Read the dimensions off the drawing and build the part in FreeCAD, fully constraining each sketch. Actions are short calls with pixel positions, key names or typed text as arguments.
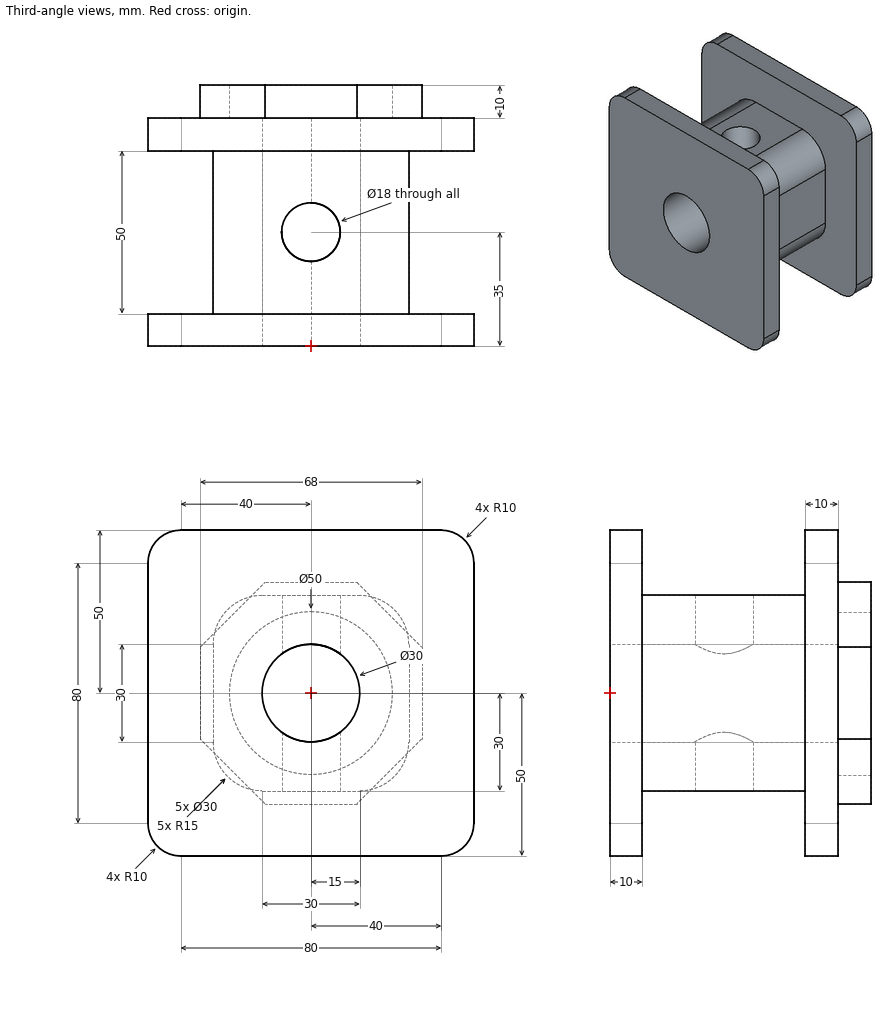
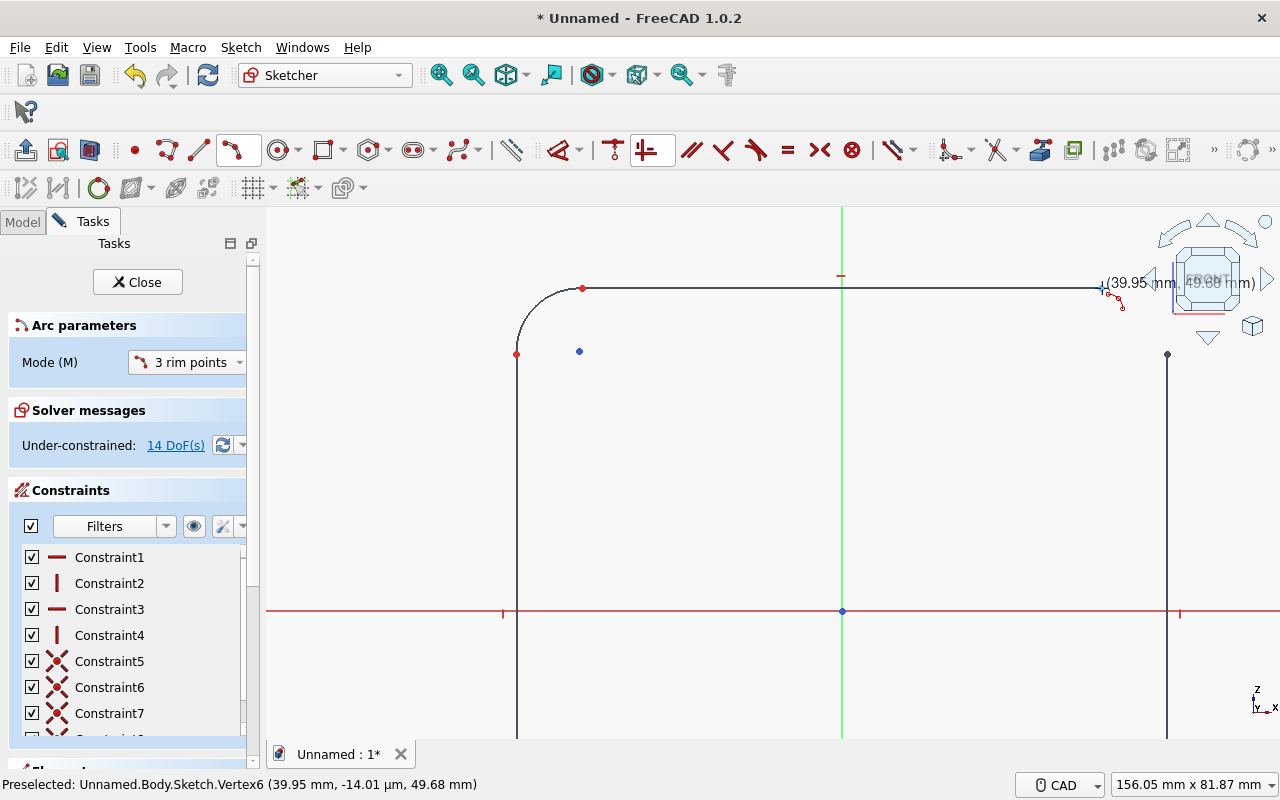
scroll(537, 305, down, 3)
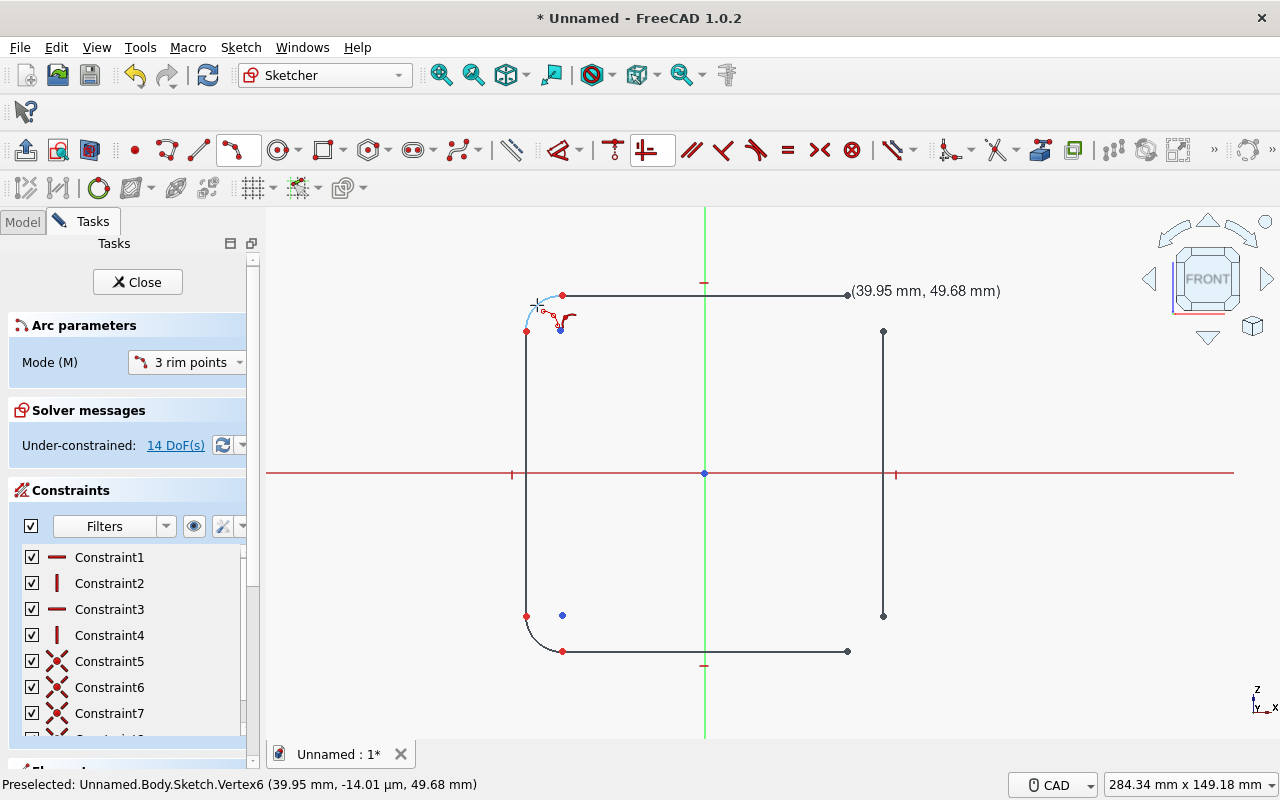
click(883, 332)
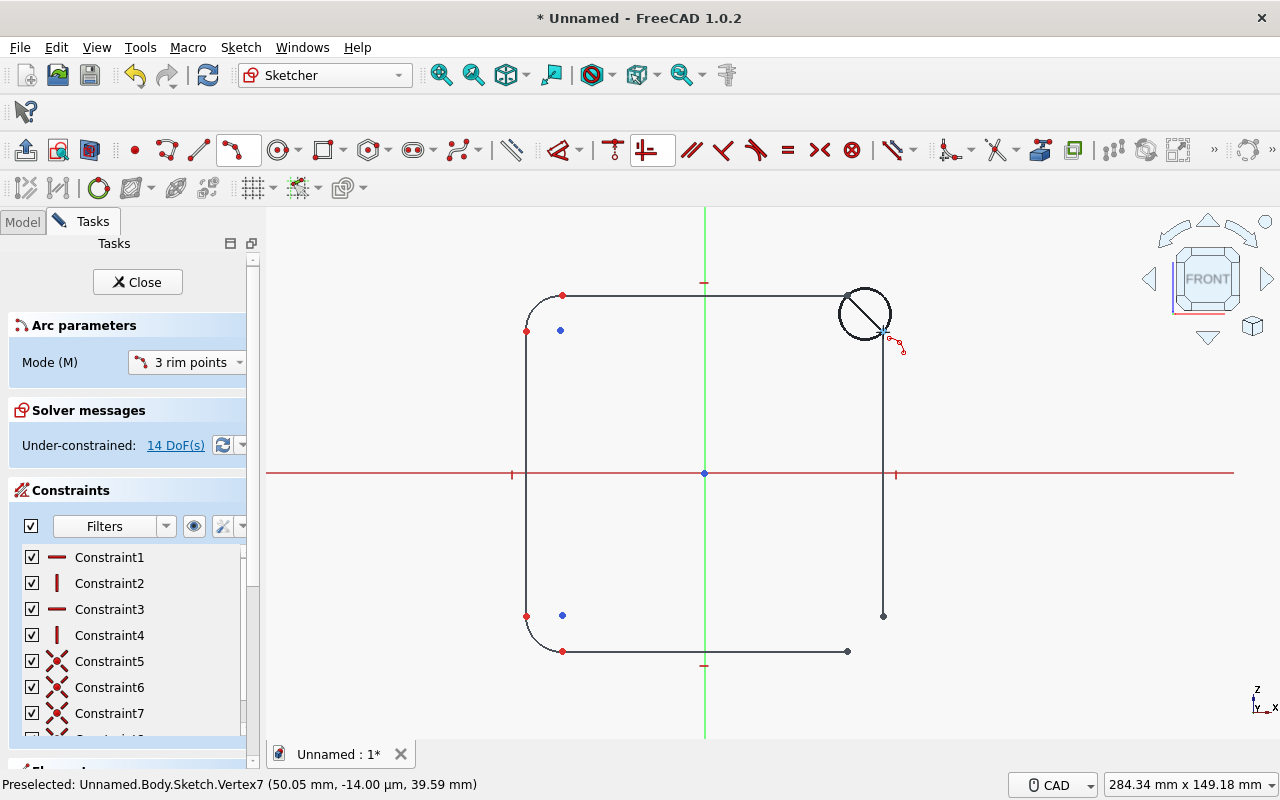
scroll(872, 305, up, 3)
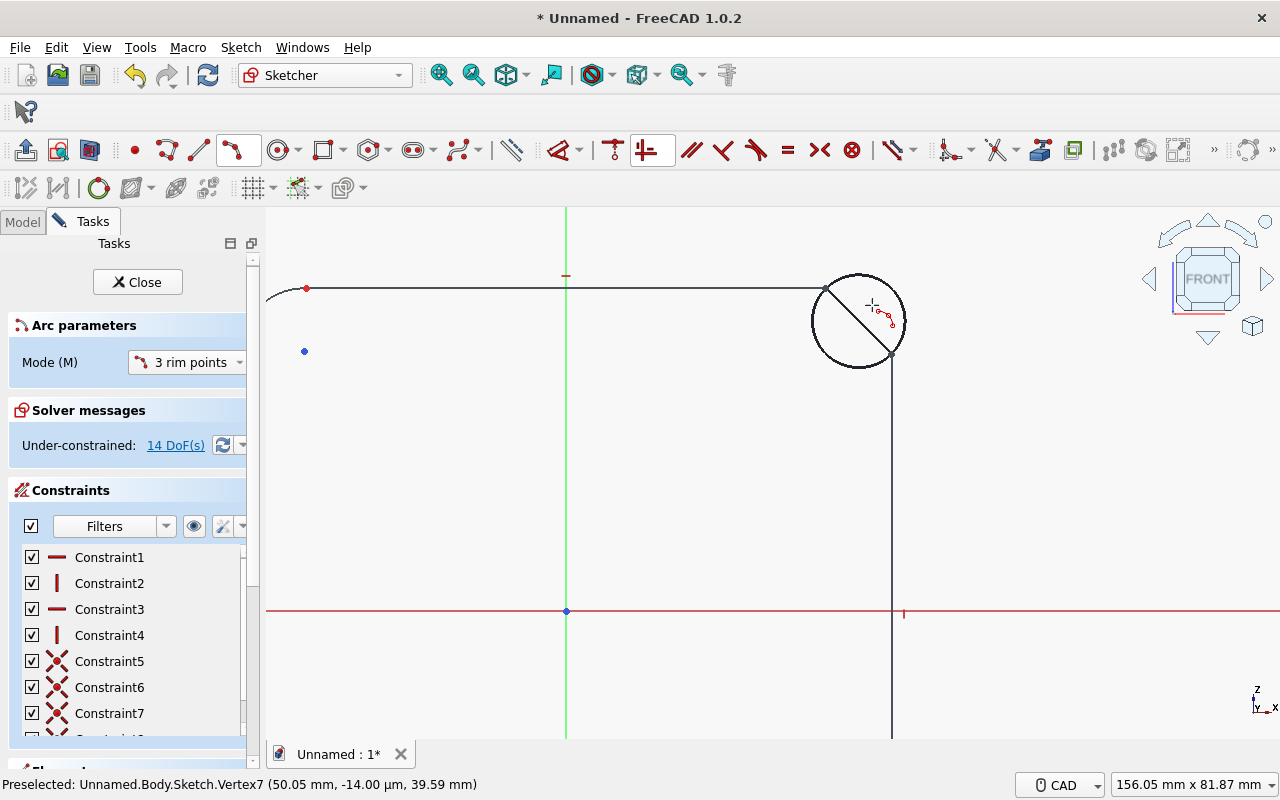
click(872, 305)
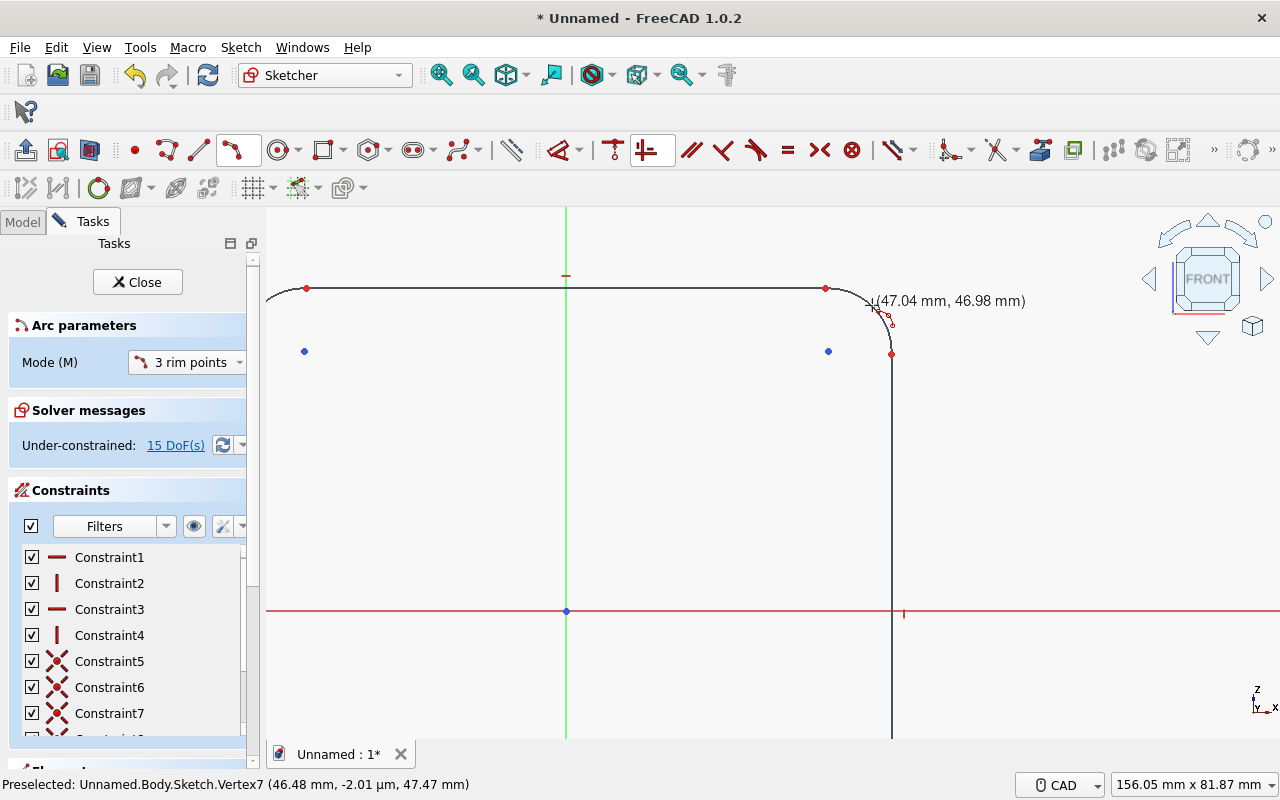
scroll(873, 305, down, 3)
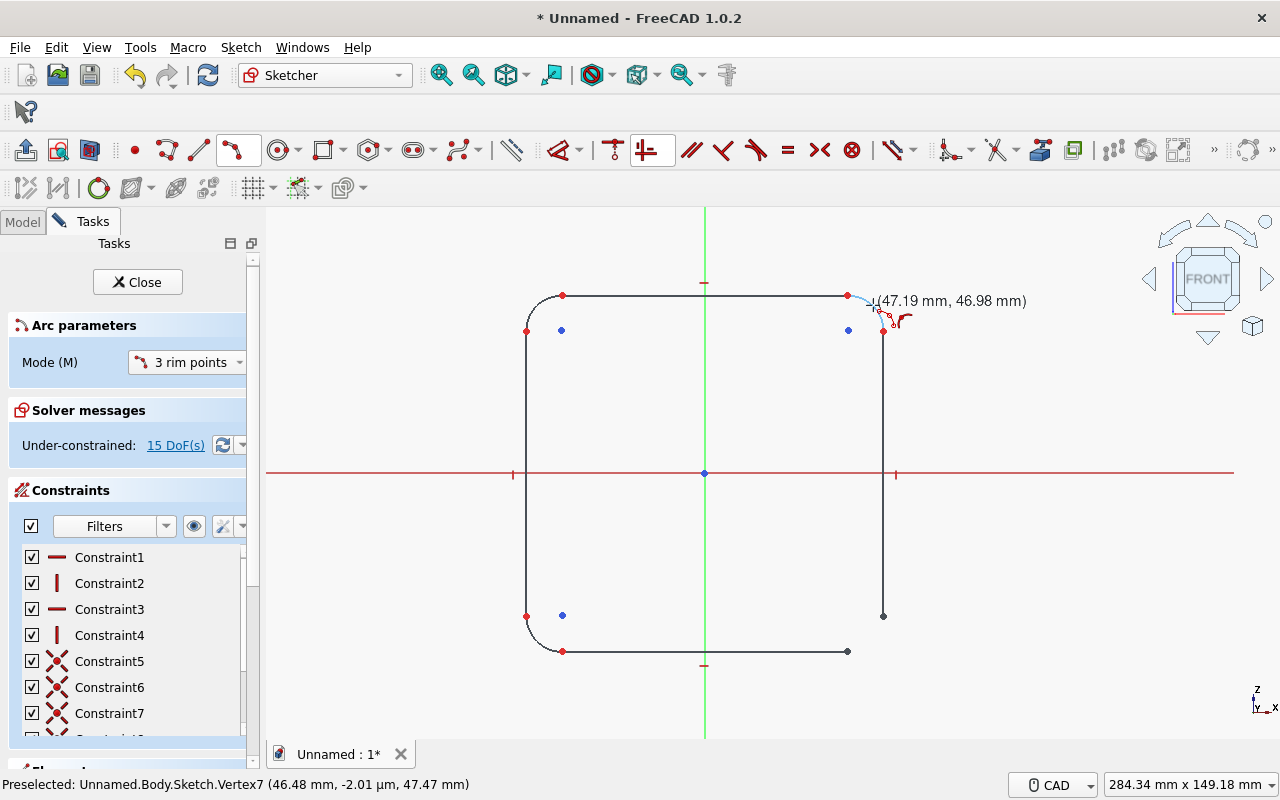
click(883, 617)
click(847, 652)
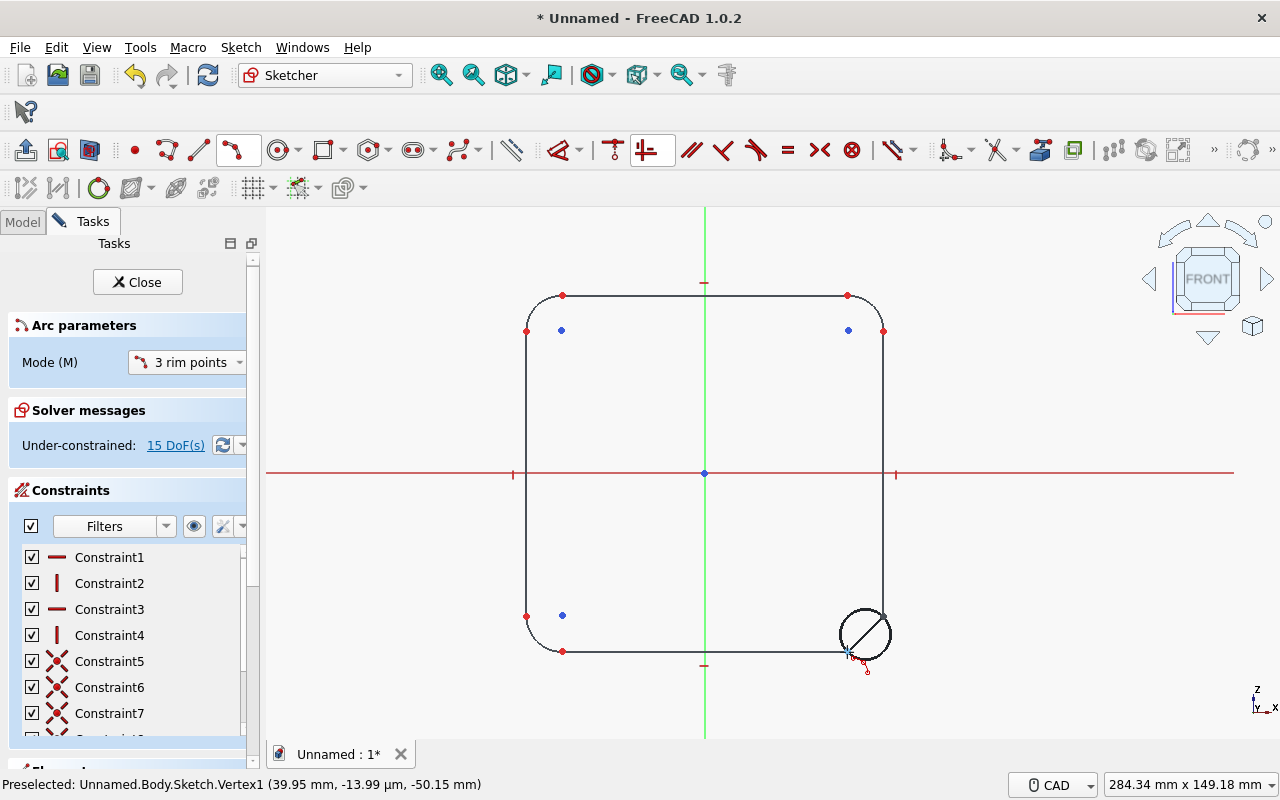
scroll(873, 641, up, 3)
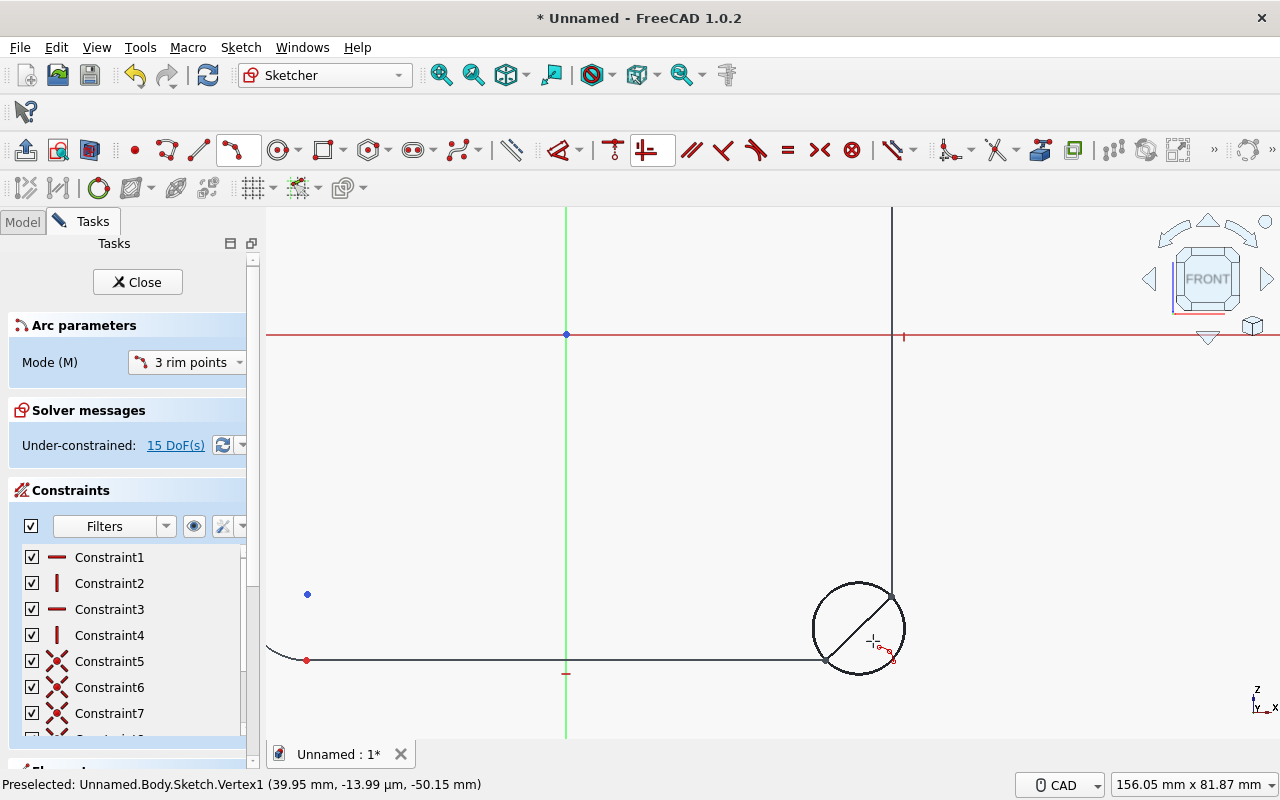
click(872, 640)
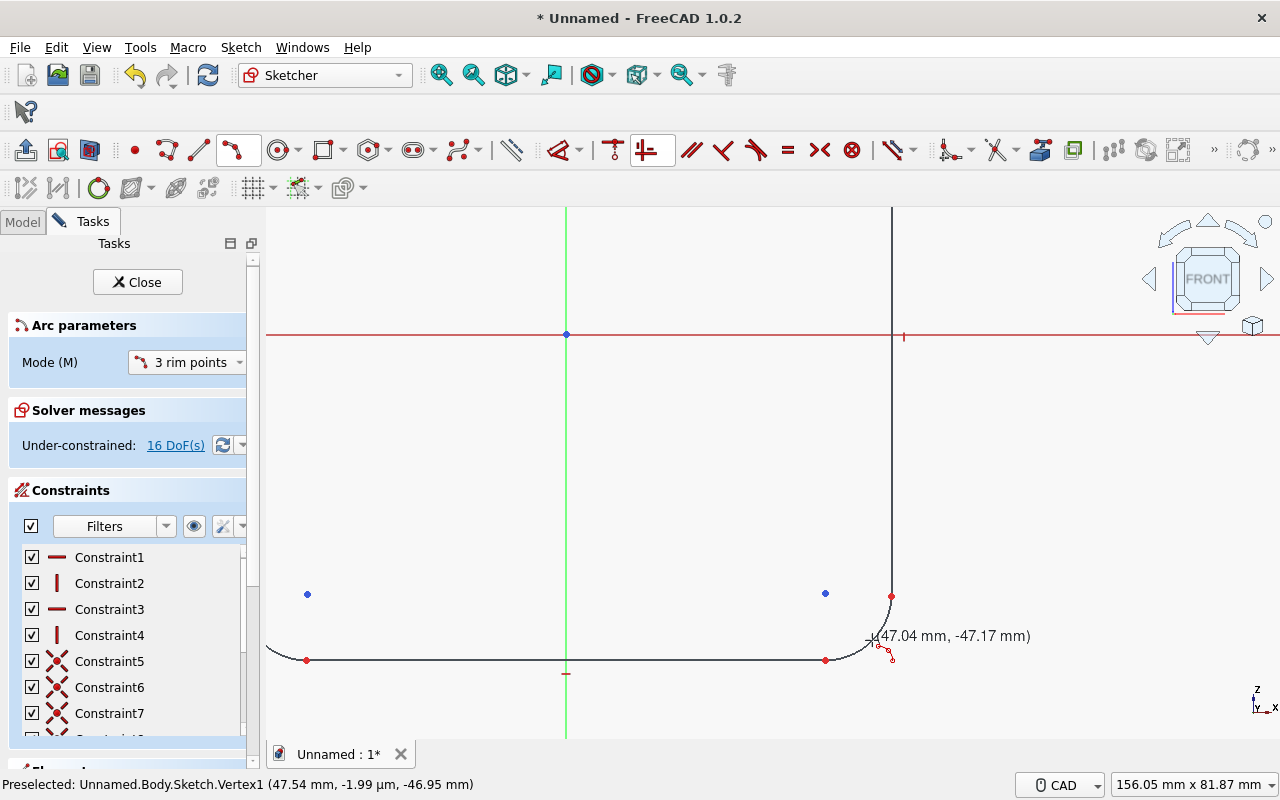
click(278, 150)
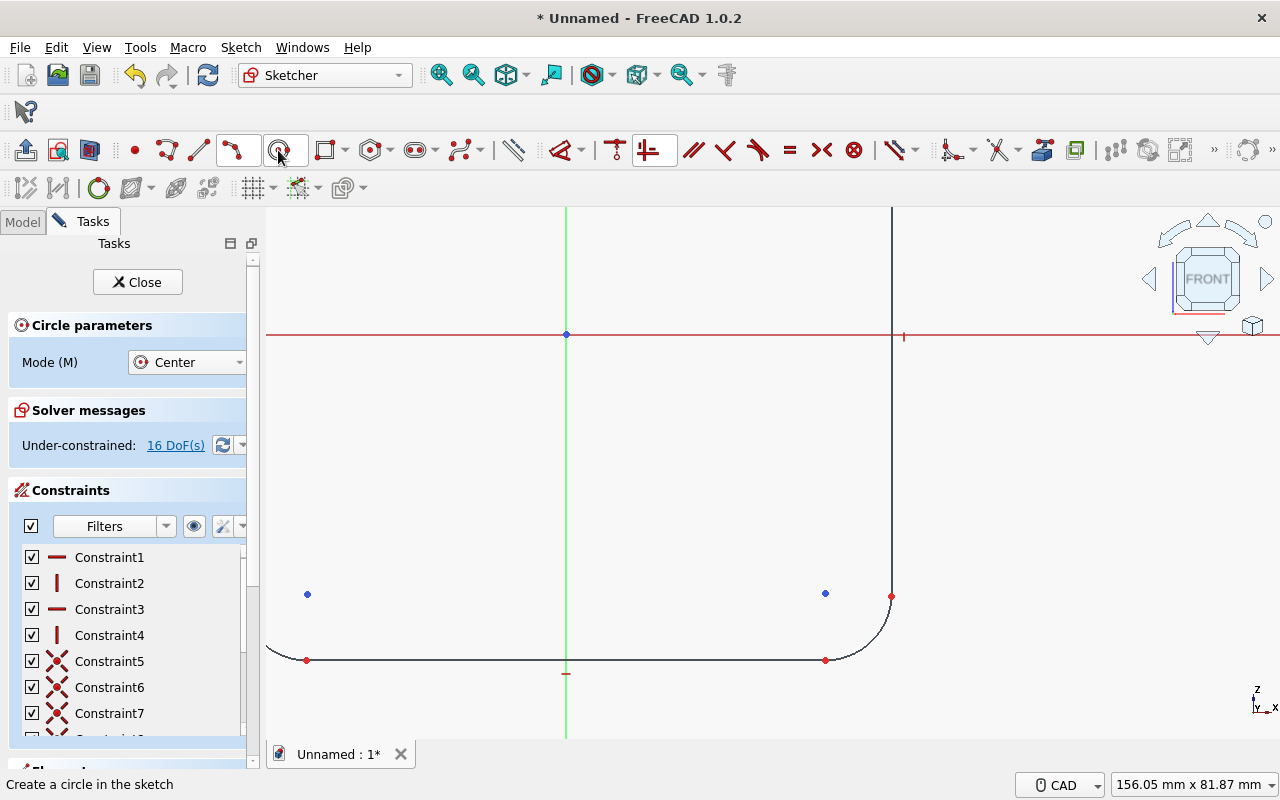
click(566, 335)
move(635, 266)